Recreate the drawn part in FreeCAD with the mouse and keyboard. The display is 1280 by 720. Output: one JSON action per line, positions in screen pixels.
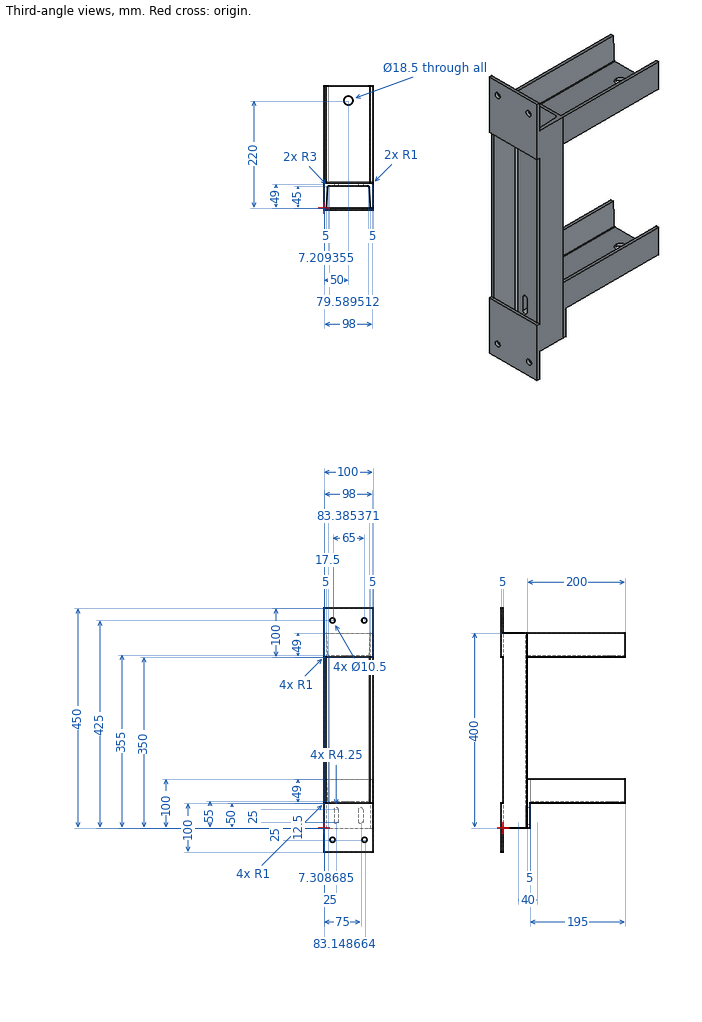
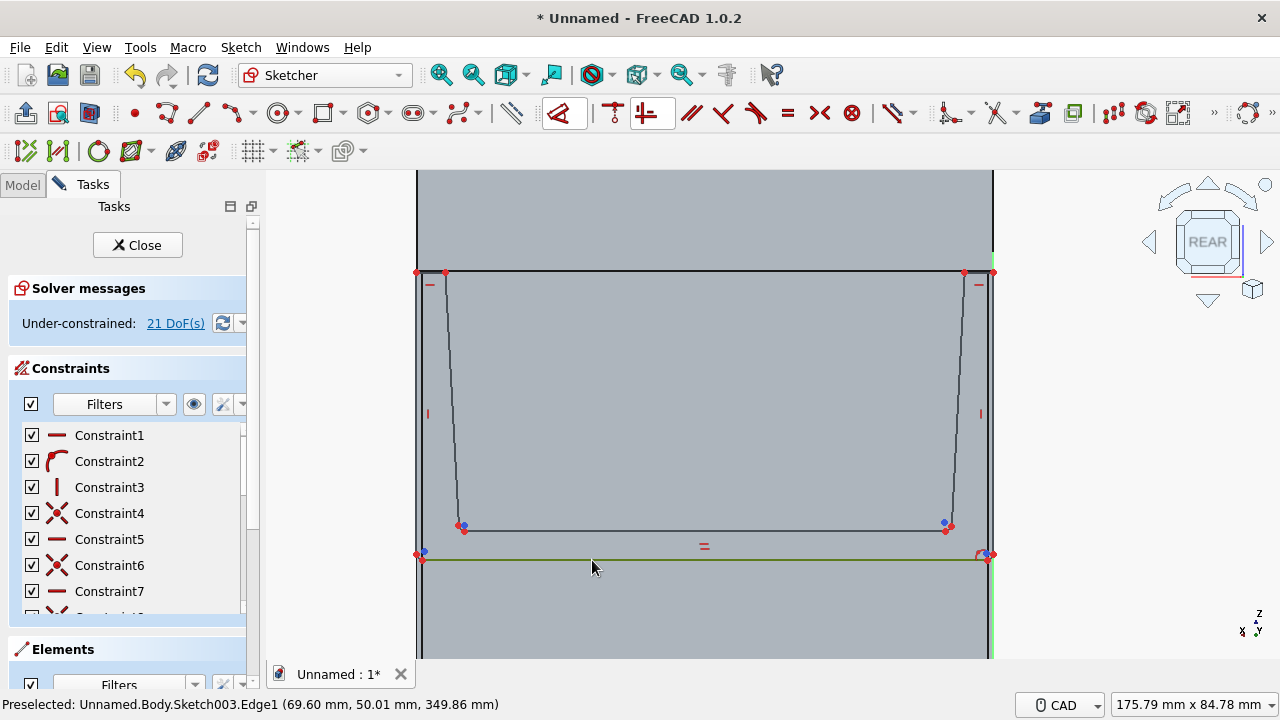
{"action": "scroll", "coordinate": [992, 558], "scroll_direction": "up", "scroll_amount": 6}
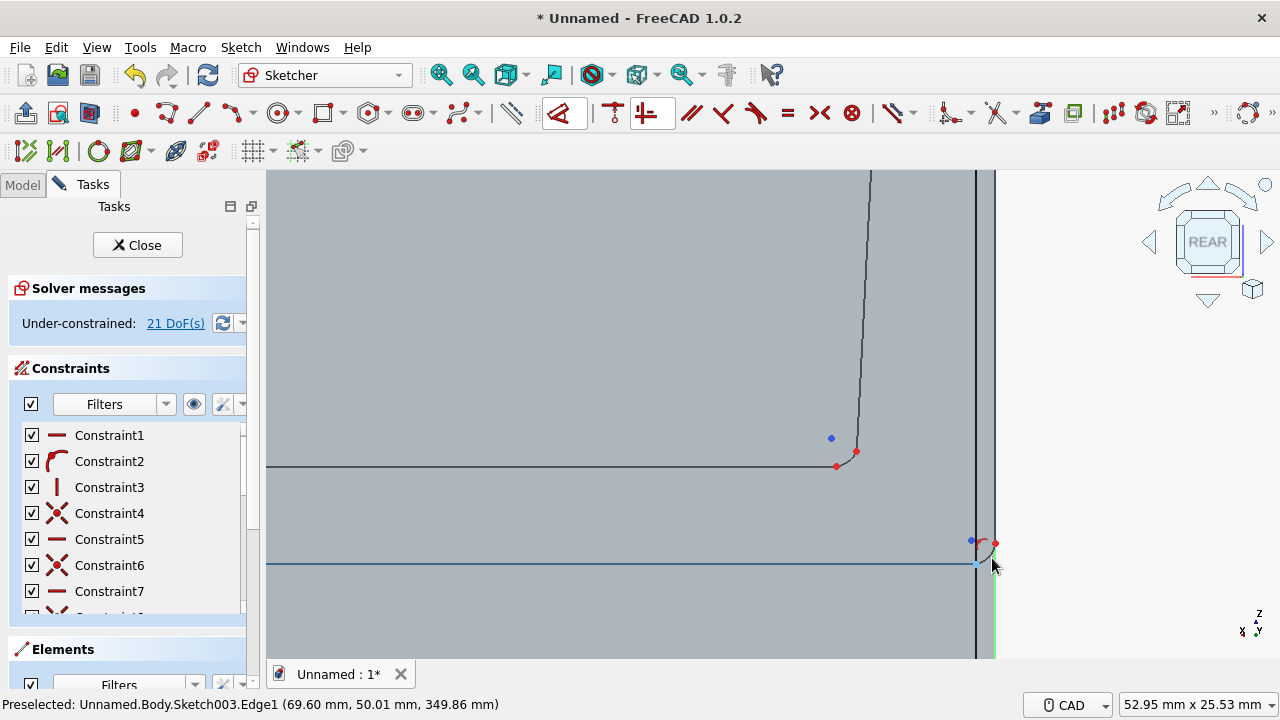
{"action": "left_click", "coordinate": [989, 557]}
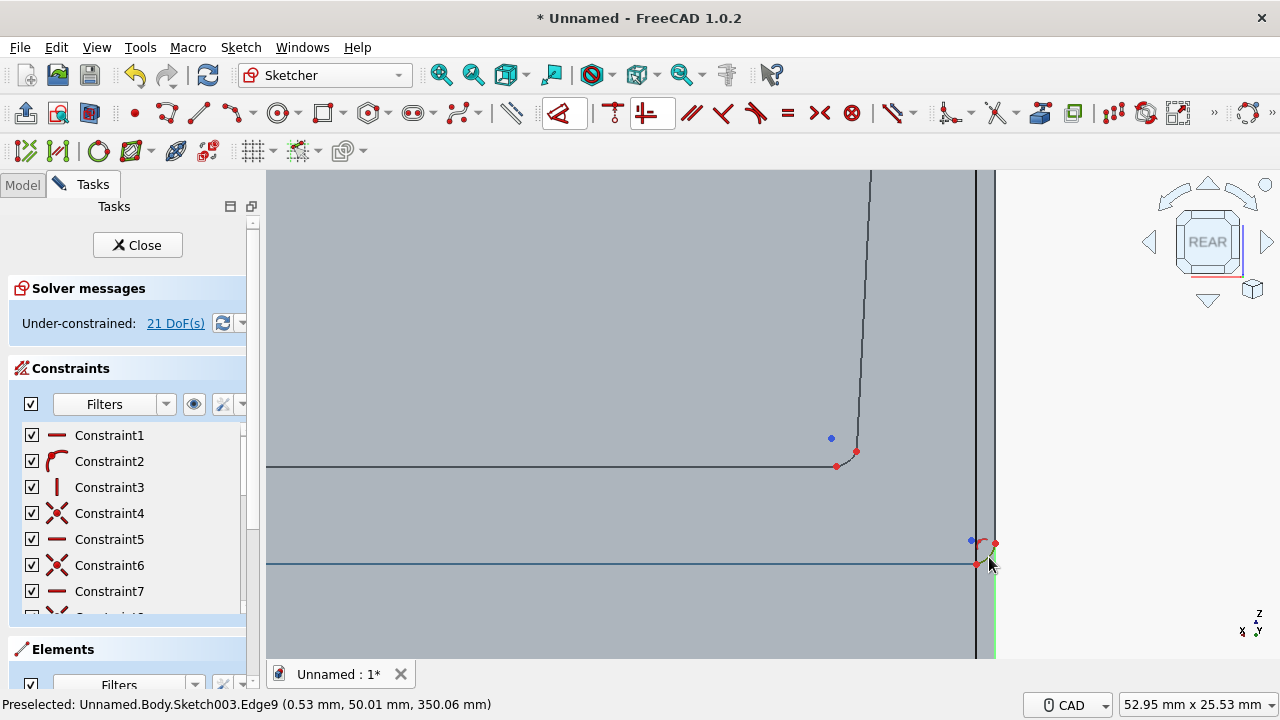
{"action": "left_click", "coordinate": [756, 114]}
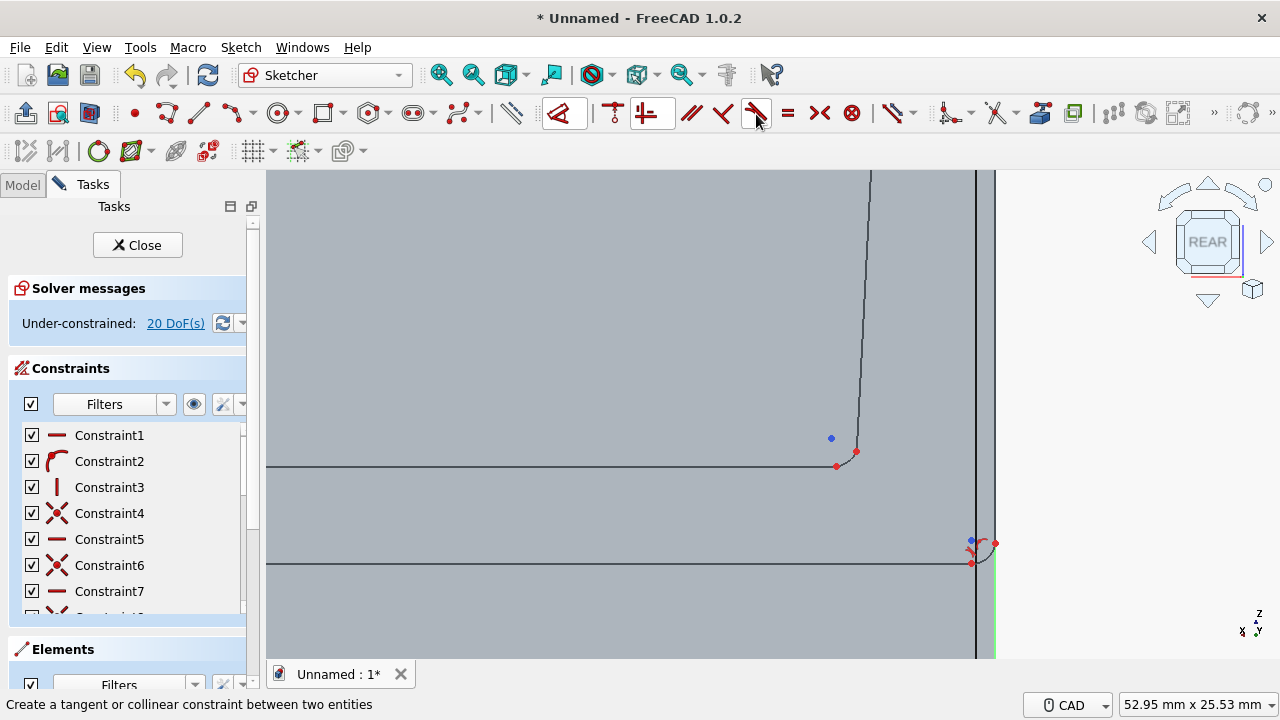
{"action": "left_click", "coordinate": [410, 564]}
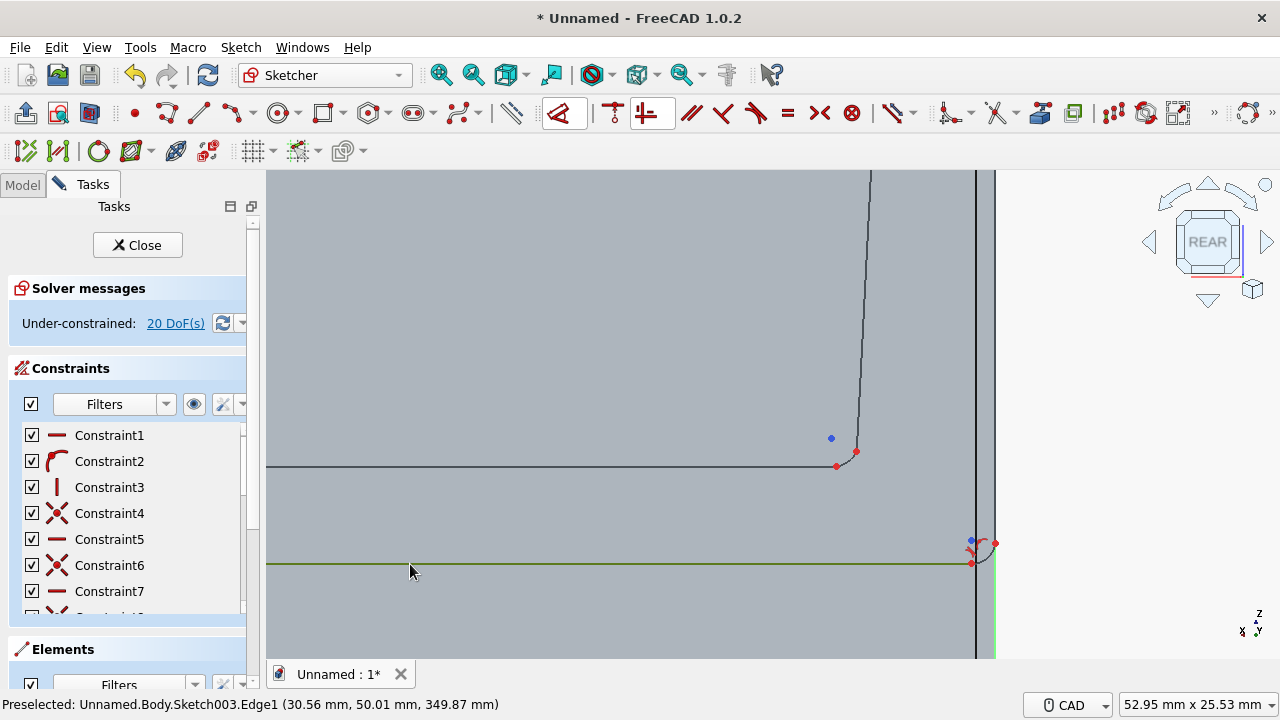
{"action": "scroll", "coordinate": [992, 557], "scroll_direction": "down", "scroll_amount": 6}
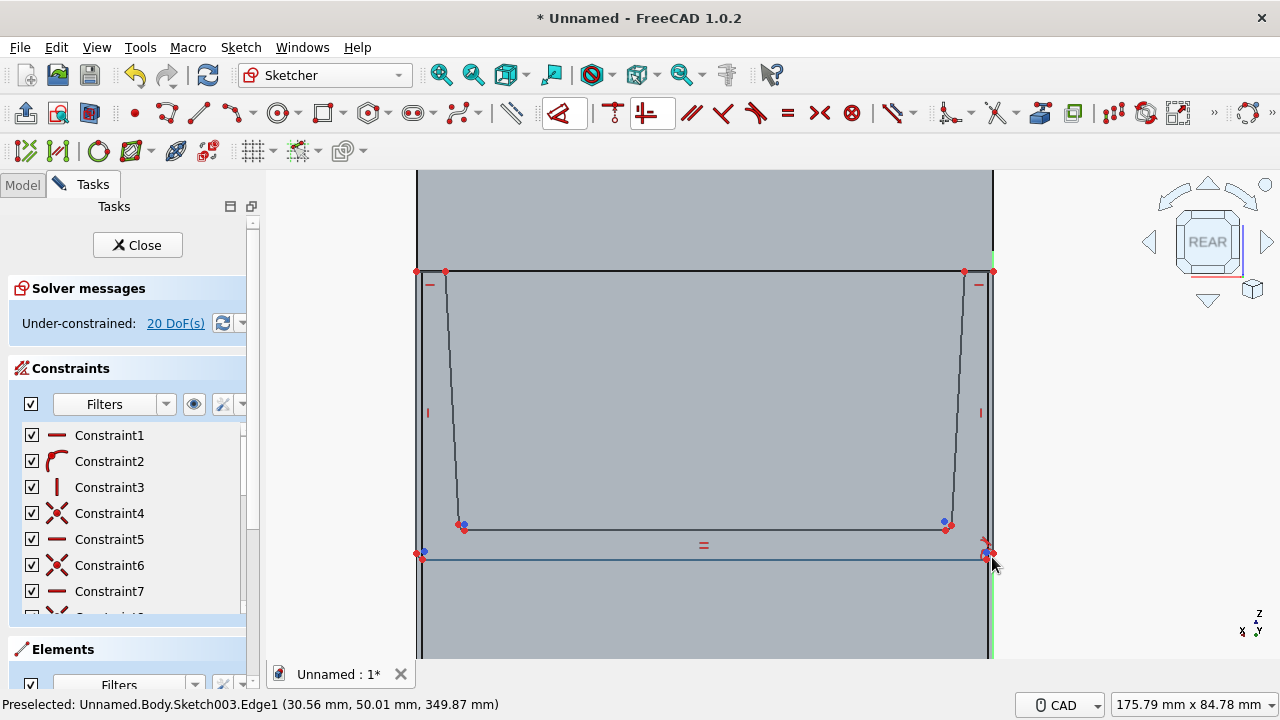
{"action": "scroll", "coordinate": [419, 557], "scroll_direction": "up", "scroll_amount": 6}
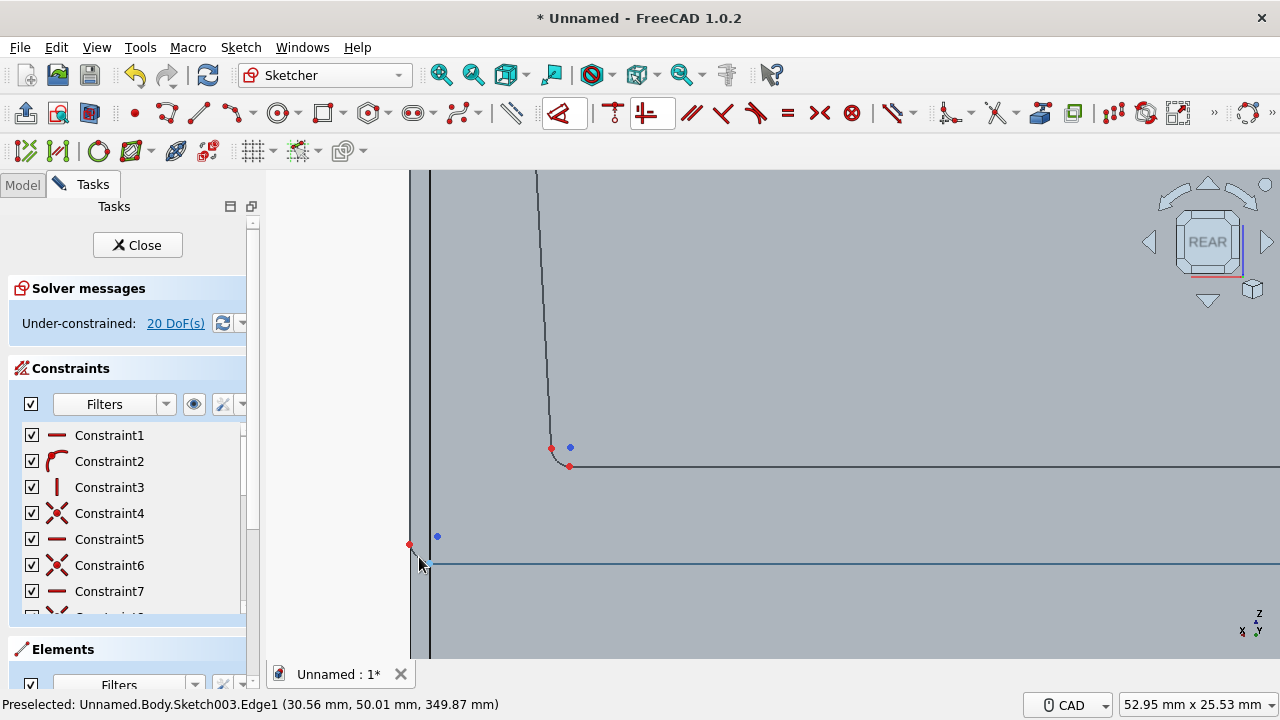
{"action": "left_click", "coordinate": [417, 557]}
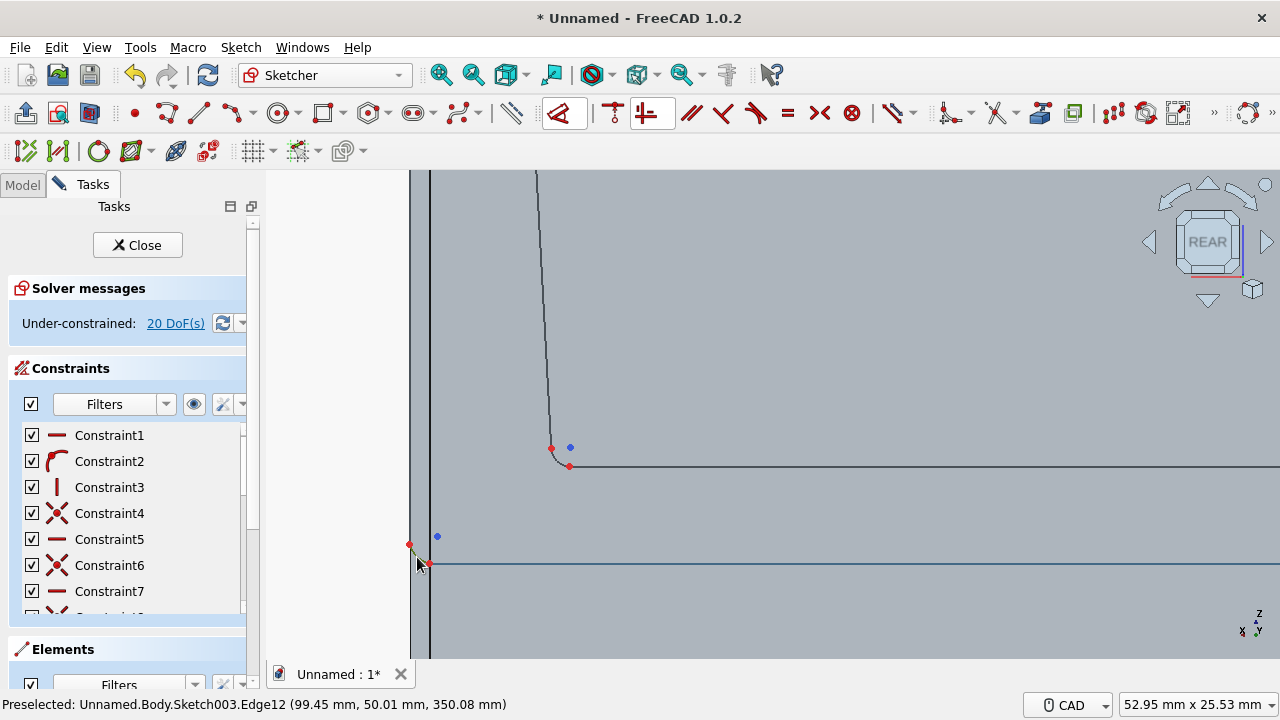
{"action": "left_click", "coordinate": [756, 114]}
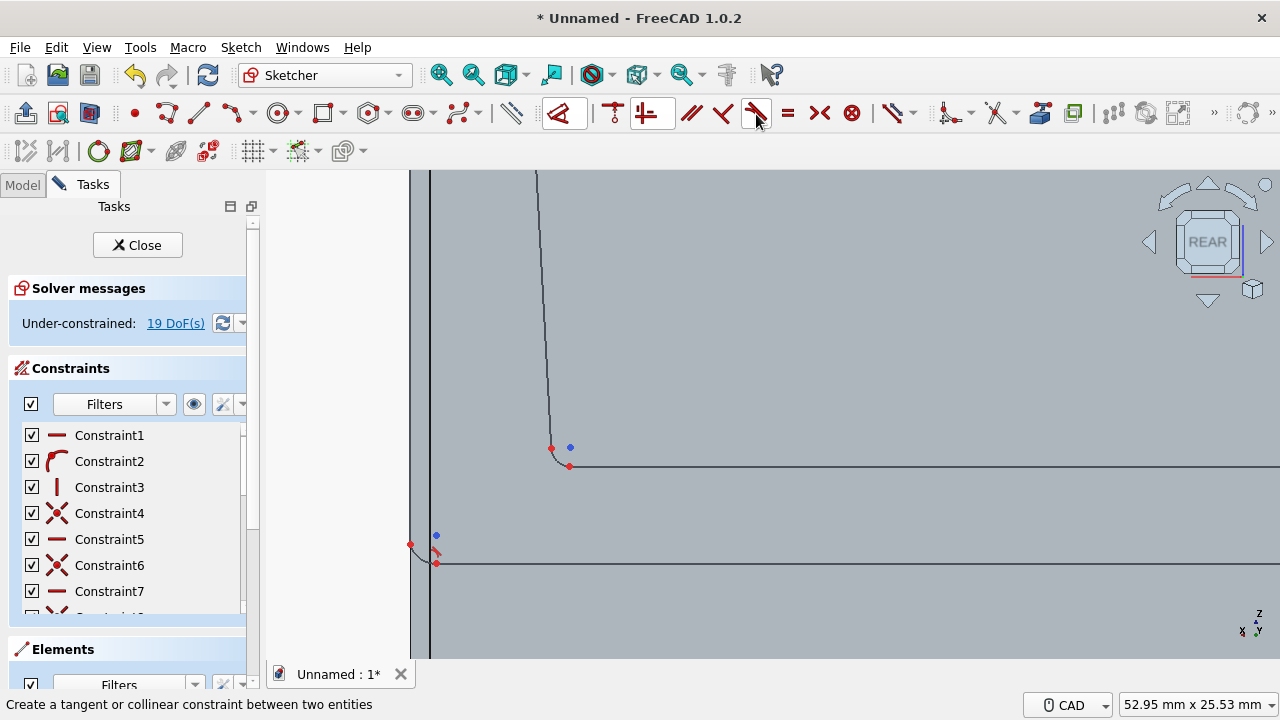
{"action": "scroll", "coordinate": [418, 557], "scroll_direction": "down", "scroll_amount": 6}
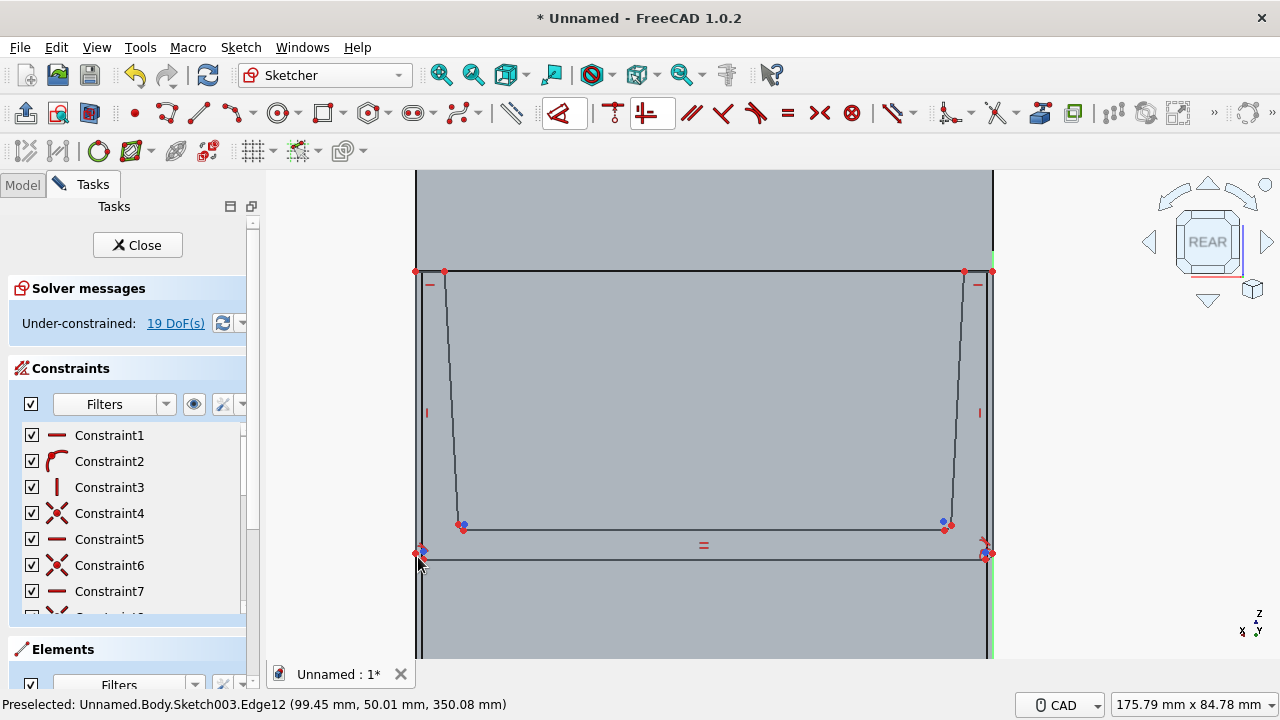
{"action": "left_click", "coordinate": [993, 469]}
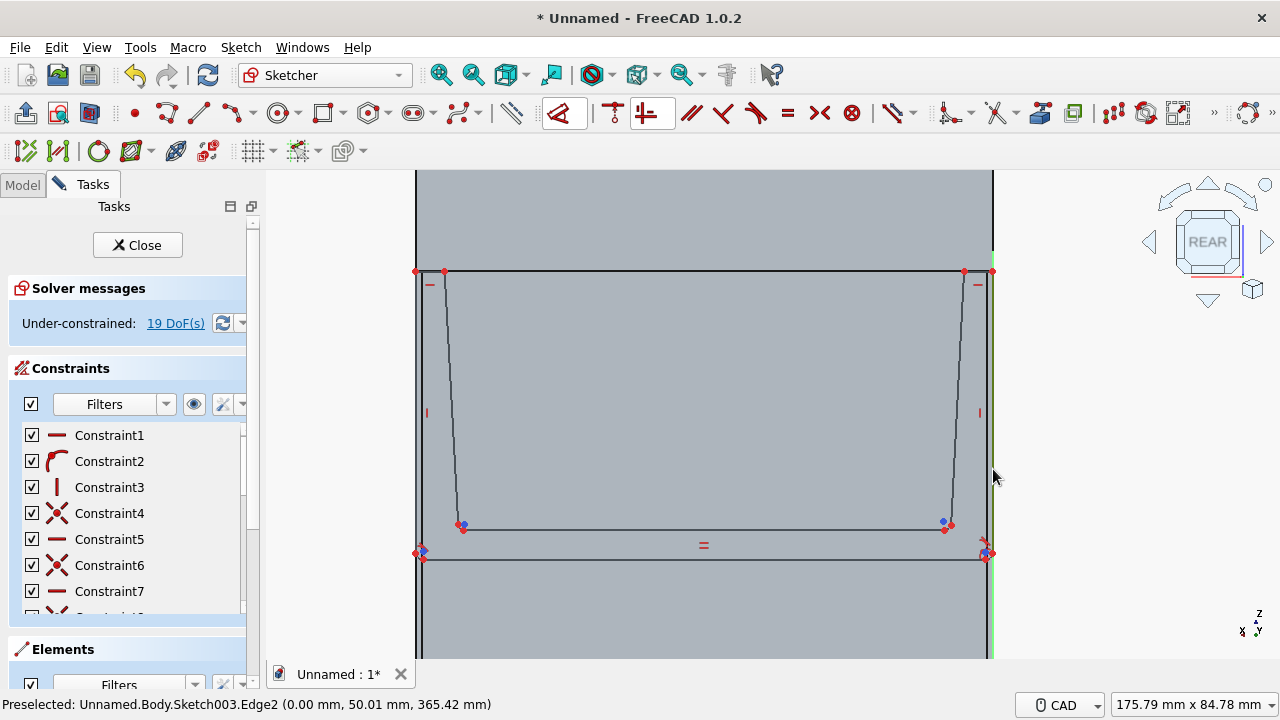
{"action": "scroll", "coordinate": [990, 558], "scroll_direction": "up", "scroll_amount": 6}